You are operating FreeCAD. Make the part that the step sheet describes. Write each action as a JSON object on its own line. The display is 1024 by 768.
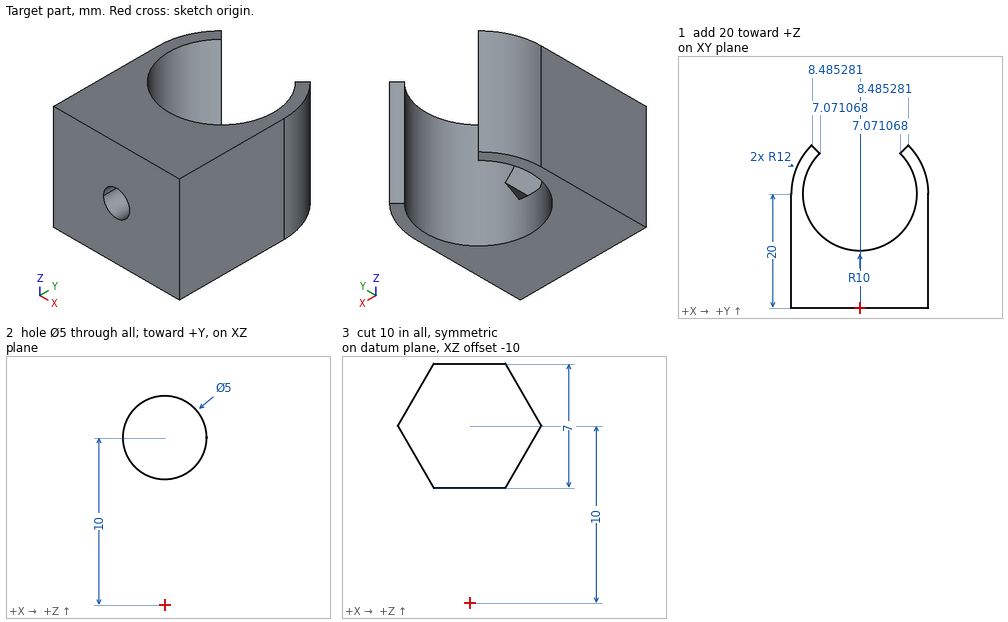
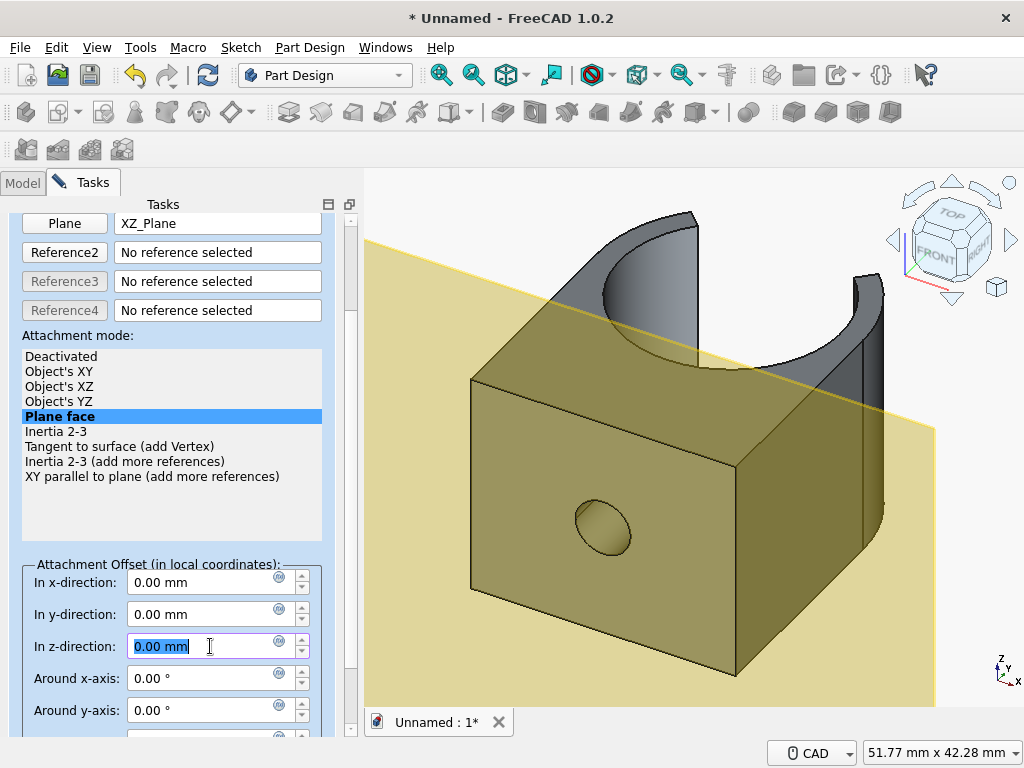
{"action": "type", "text": "-10"}
{"action": "key", "text": "Tab"}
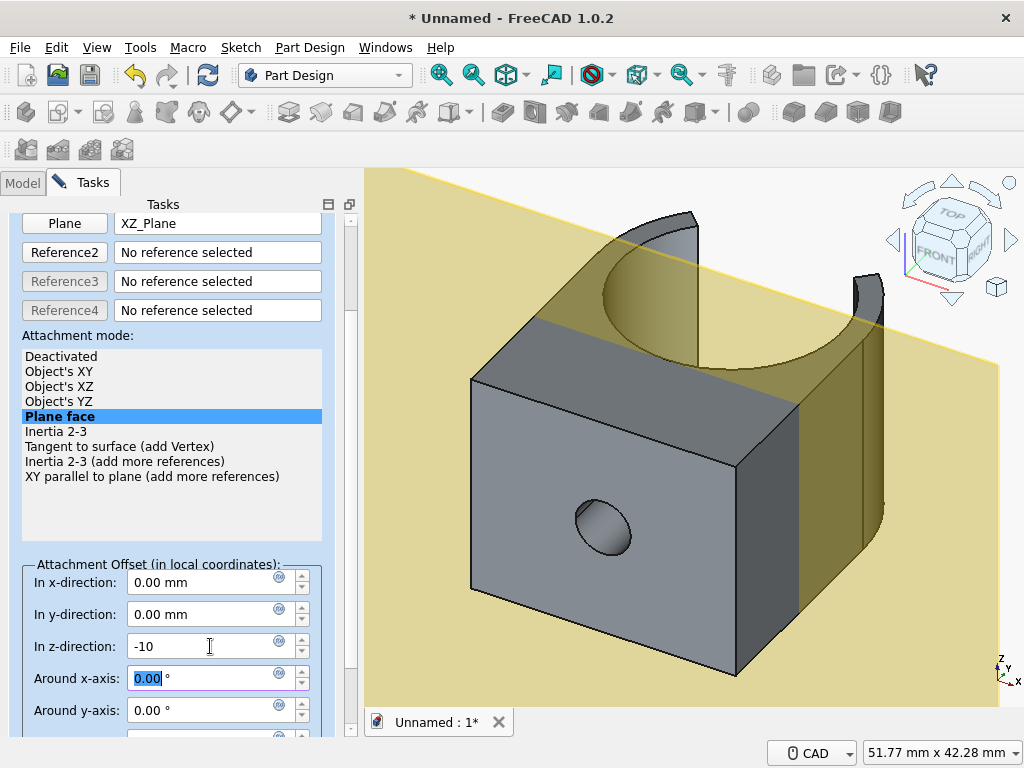
{"action": "scroll", "coordinate": [351, 475], "scroll_direction": "up", "scroll_amount": 3}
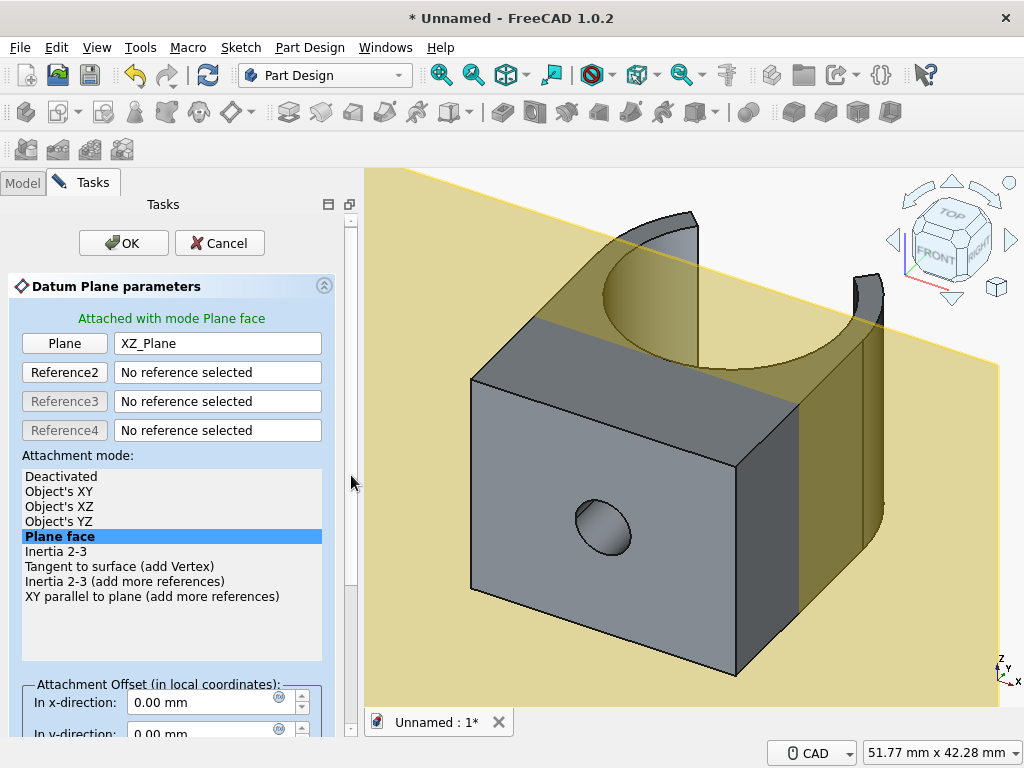
{"action": "left_click", "coordinate": [124, 243]}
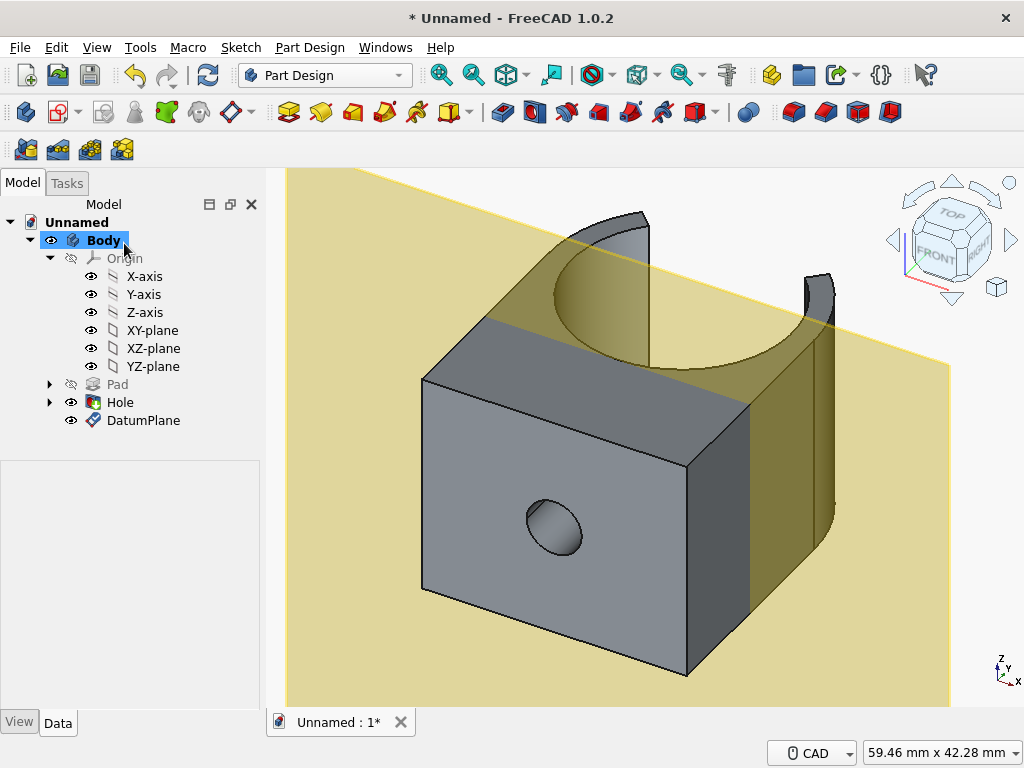
{"action": "left_click", "coordinate": [116, 420]}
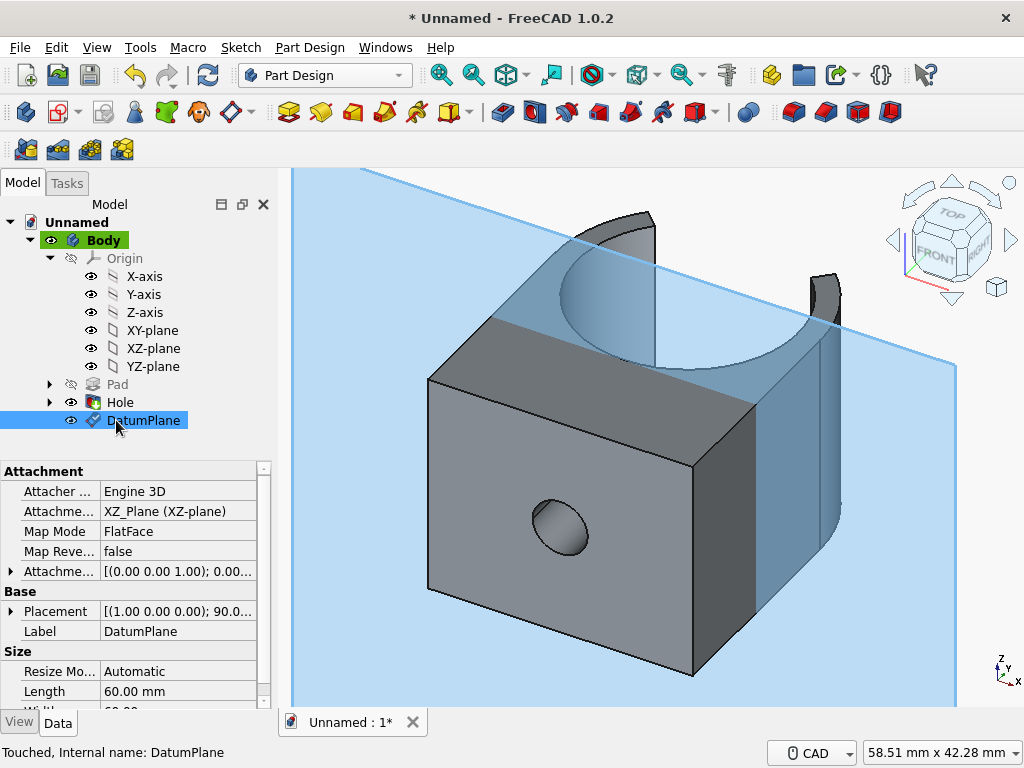
{"action": "left_click", "coordinate": [58, 112]}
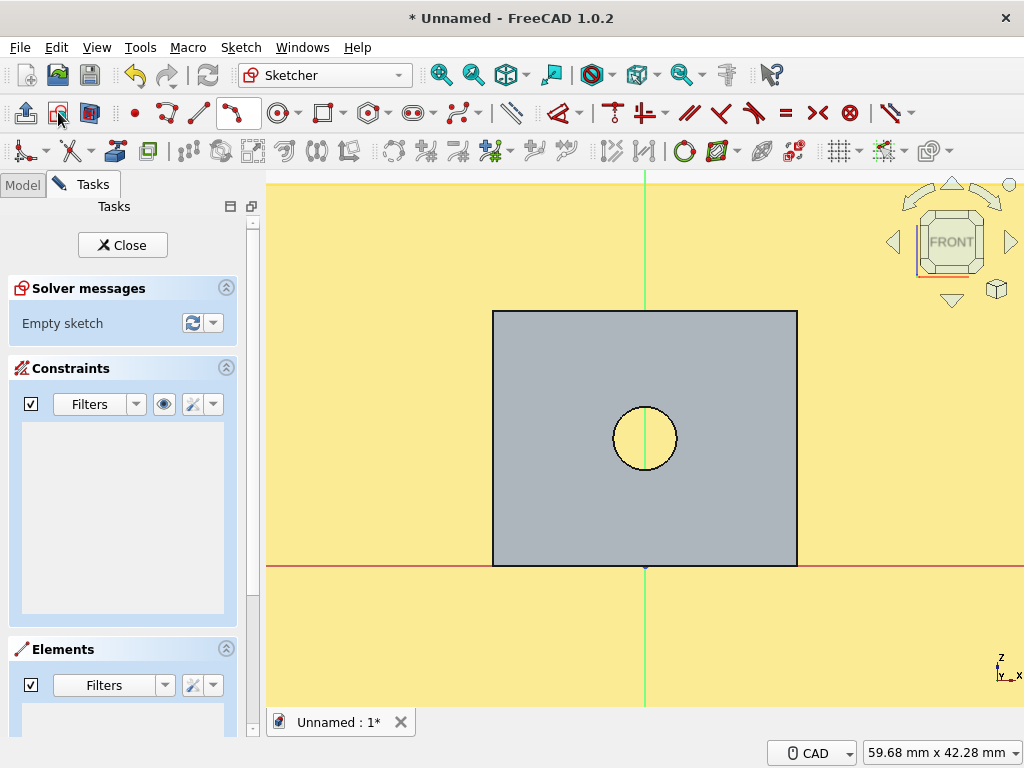
{"action": "left_click", "coordinate": [90, 114]}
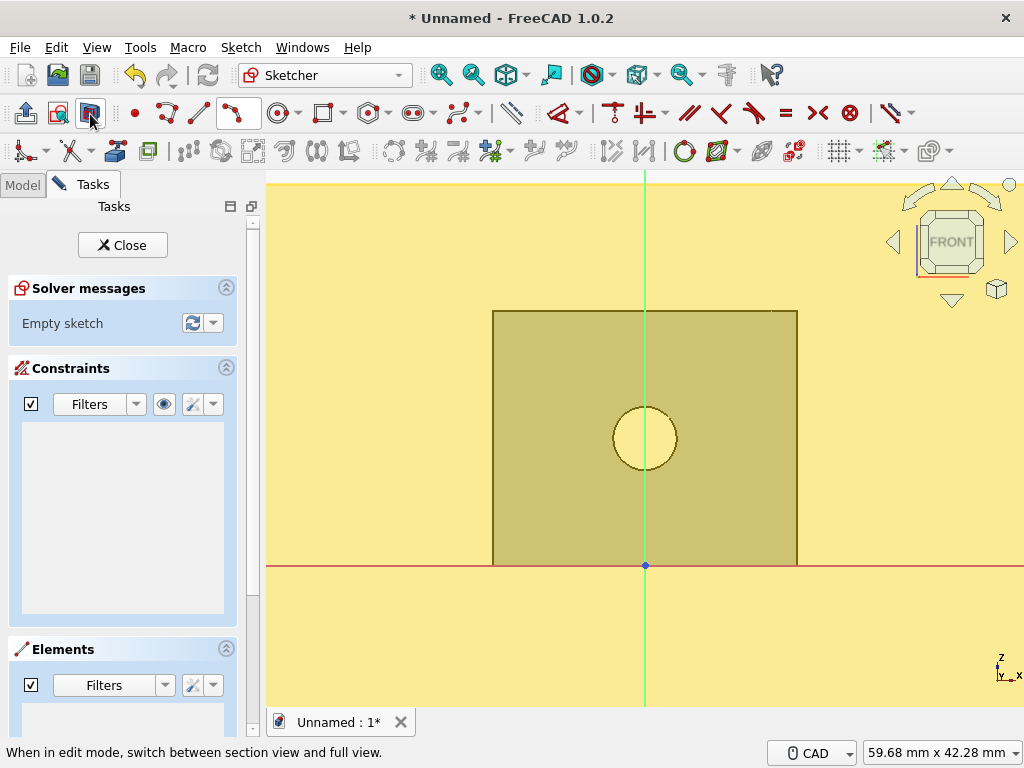
{"action": "scroll", "coordinate": [728, 530], "scroll_direction": "up", "scroll_amount": 3}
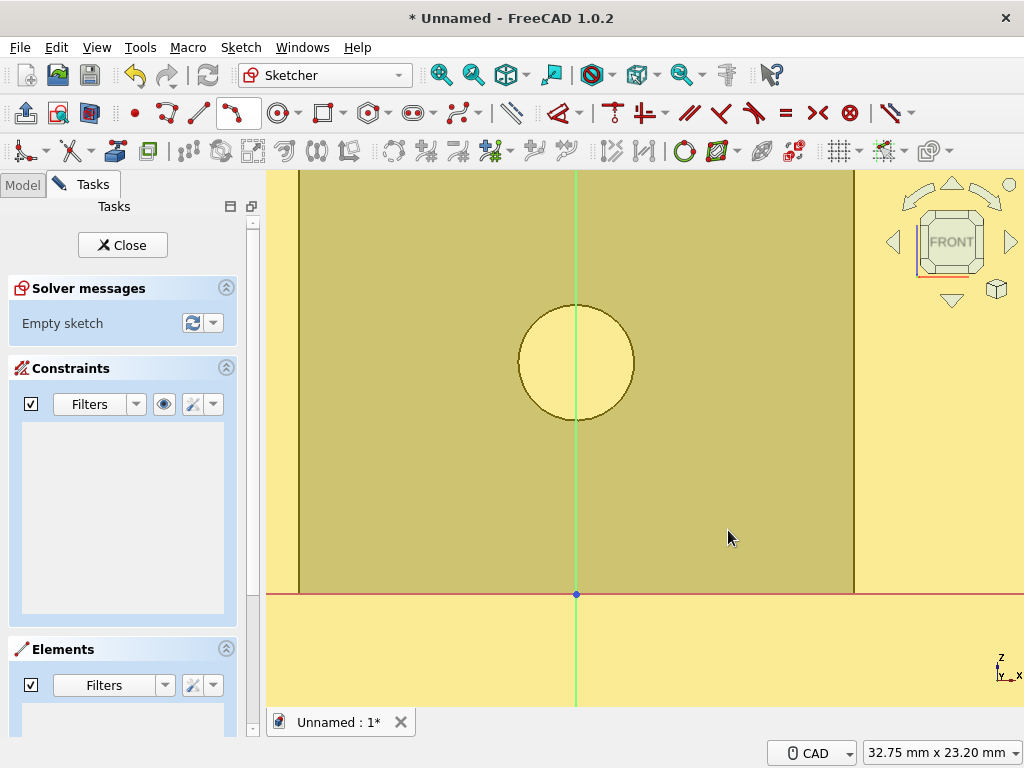
{"action": "left_click", "coordinate": [368, 114]}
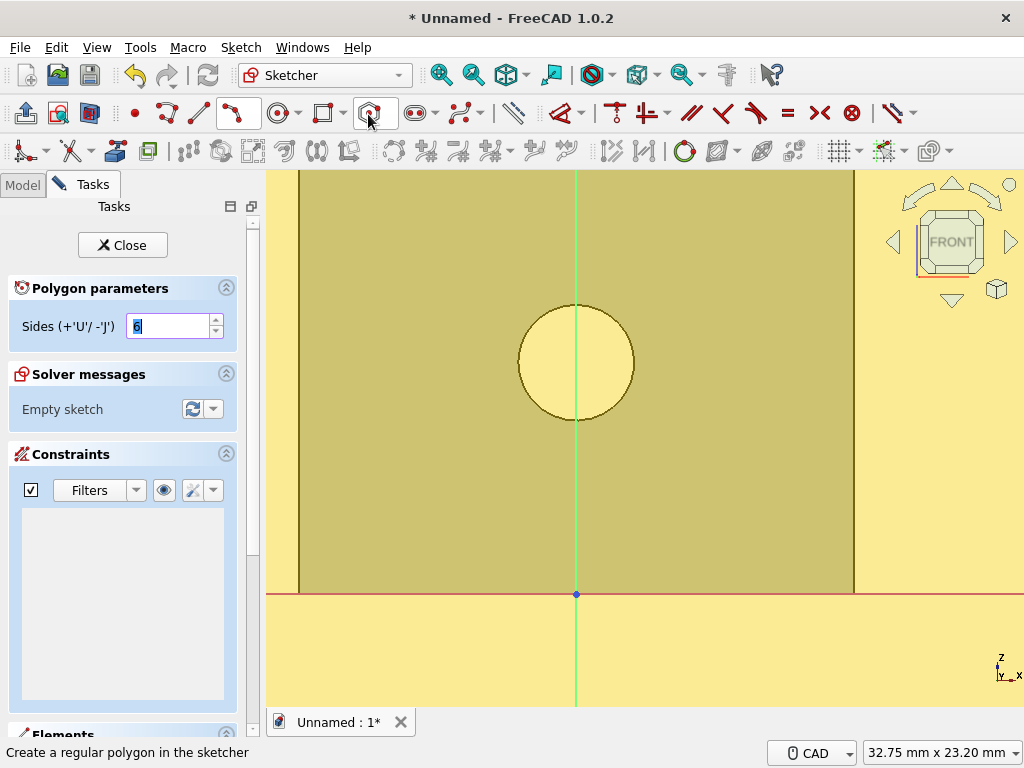
{"action": "left_click", "coordinate": [576, 363]}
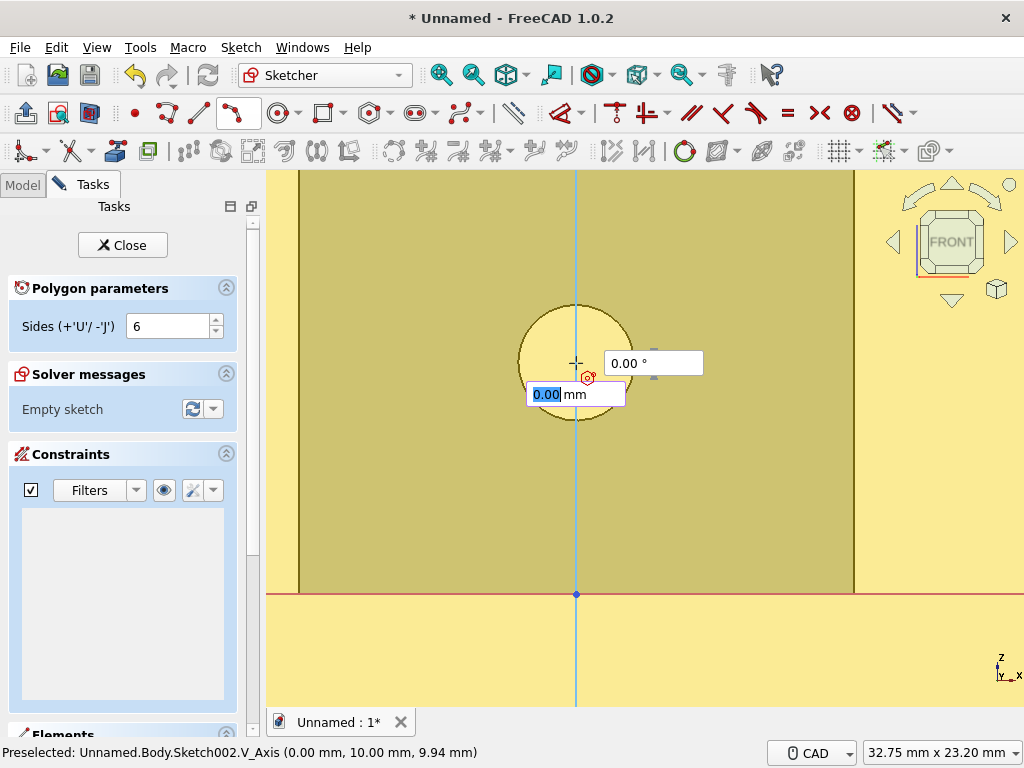
{"action": "left_click", "coordinate": [483, 363]}
{"action": "right_click", "coordinate": [483, 363]}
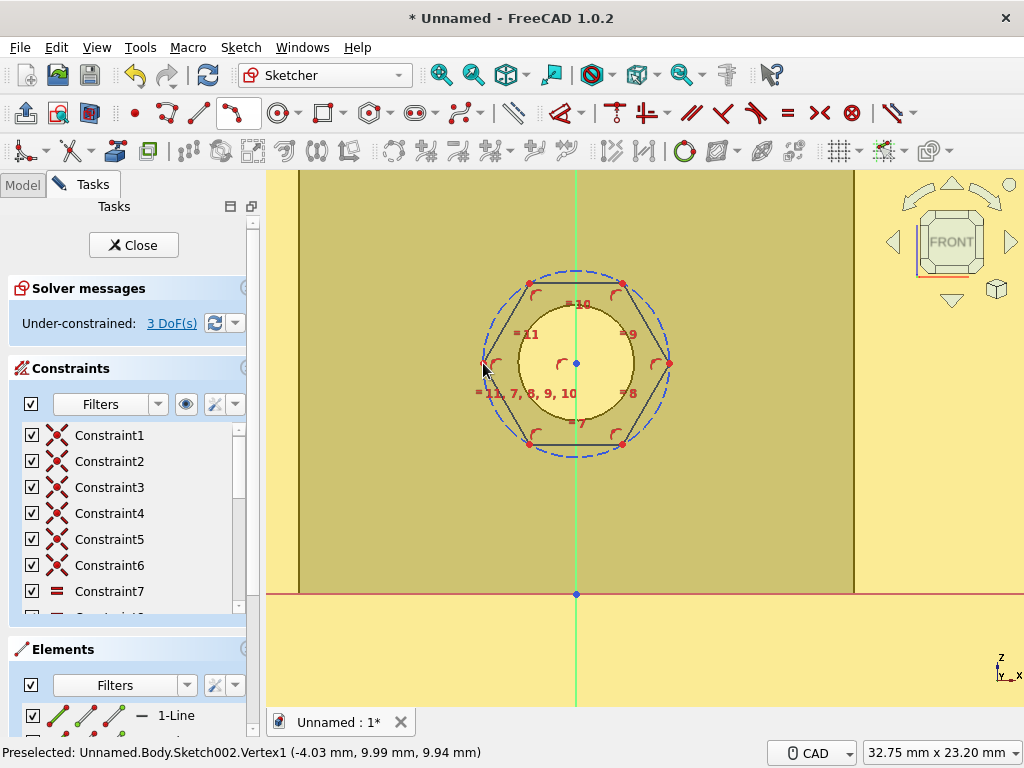
{"action": "scroll", "coordinate": [558, 445], "scroll_direction": "up", "scroll_amount": 2}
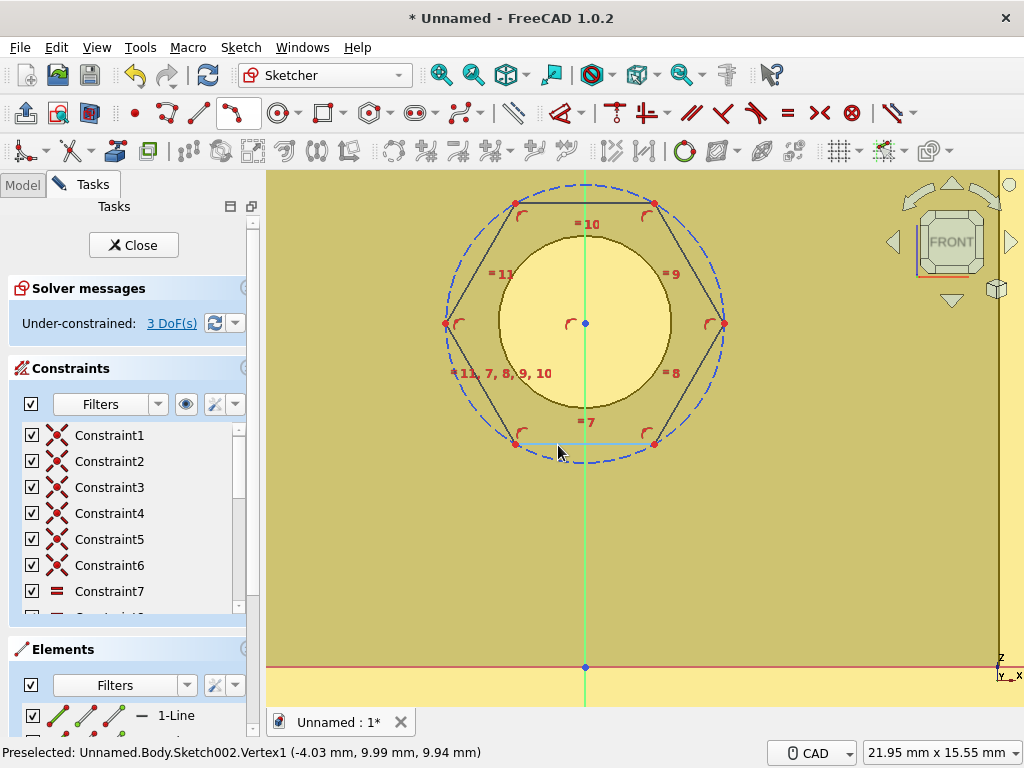
{"action": "left_click", "coordinate": [557, 444]}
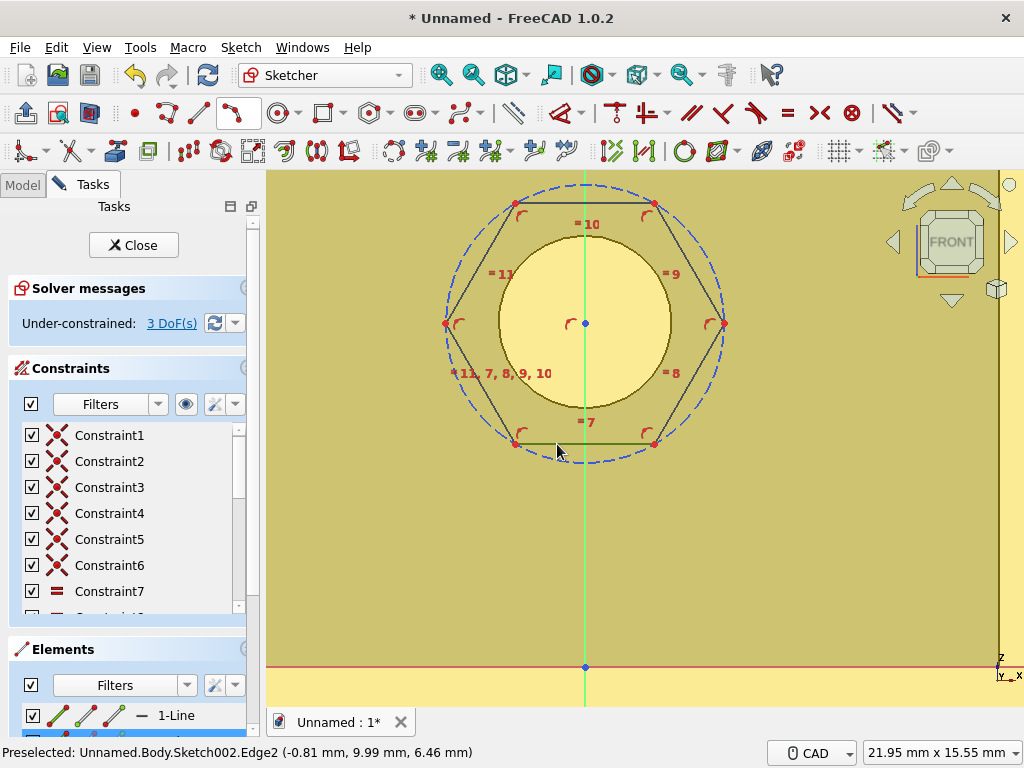
{"action": "left_click", "coordinate": [670, 114]}